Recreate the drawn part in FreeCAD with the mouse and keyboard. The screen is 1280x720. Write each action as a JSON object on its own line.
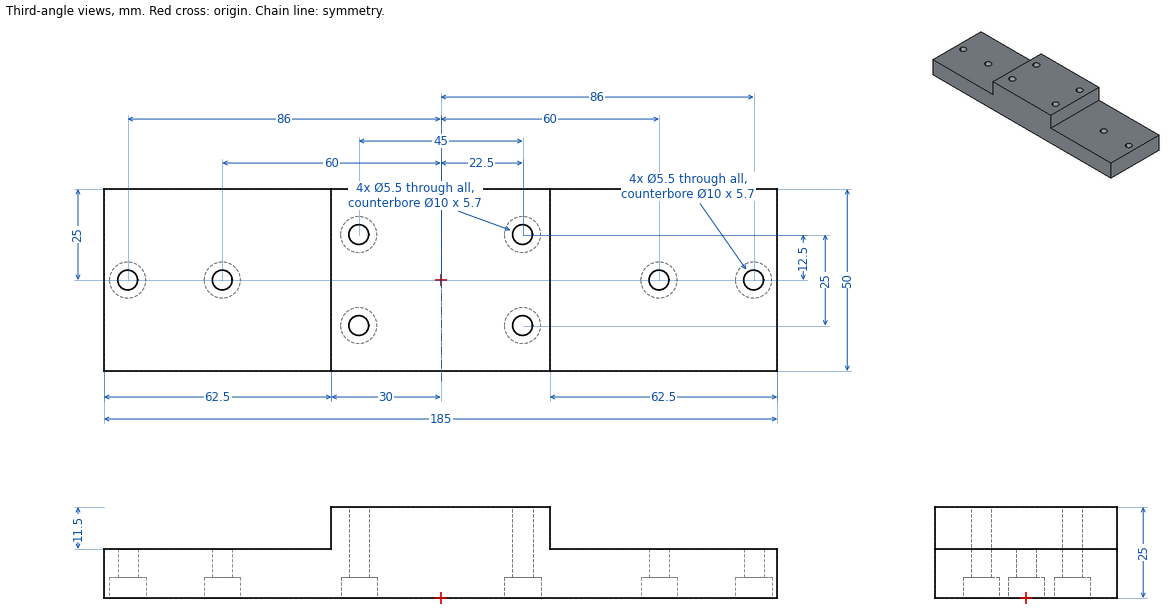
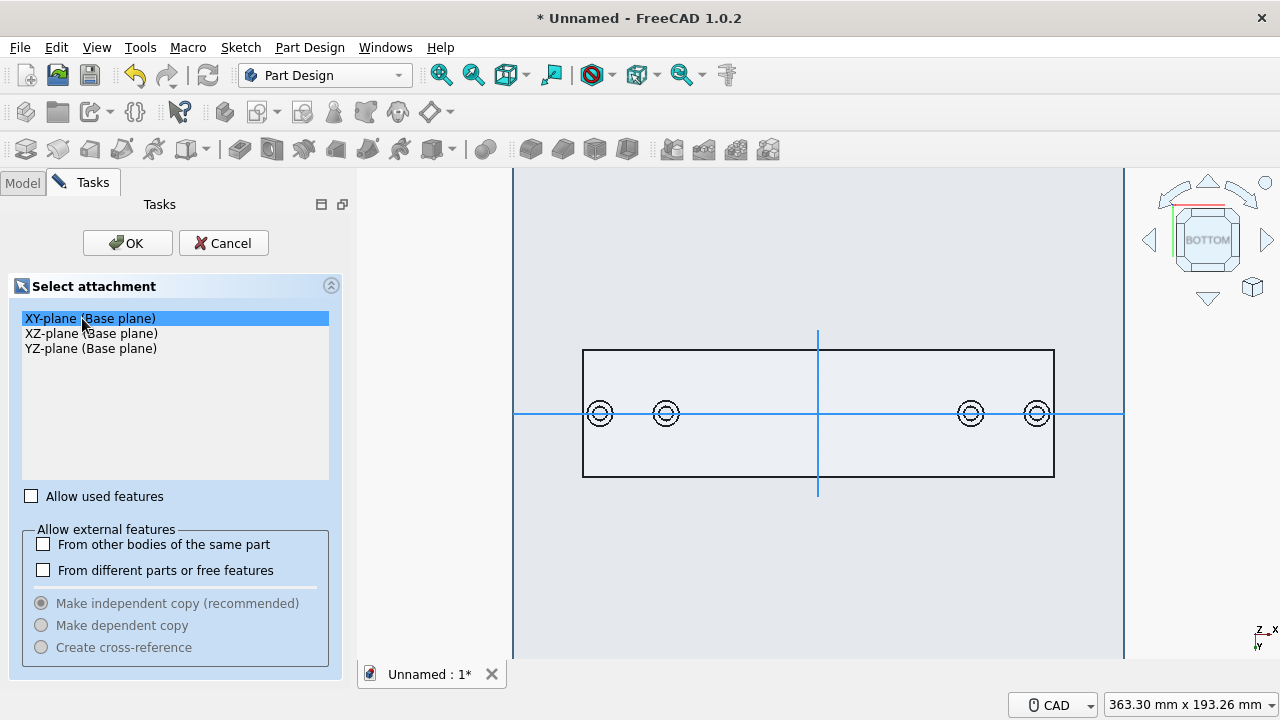
{"action": "left_click", "coordinate": [128, 243]}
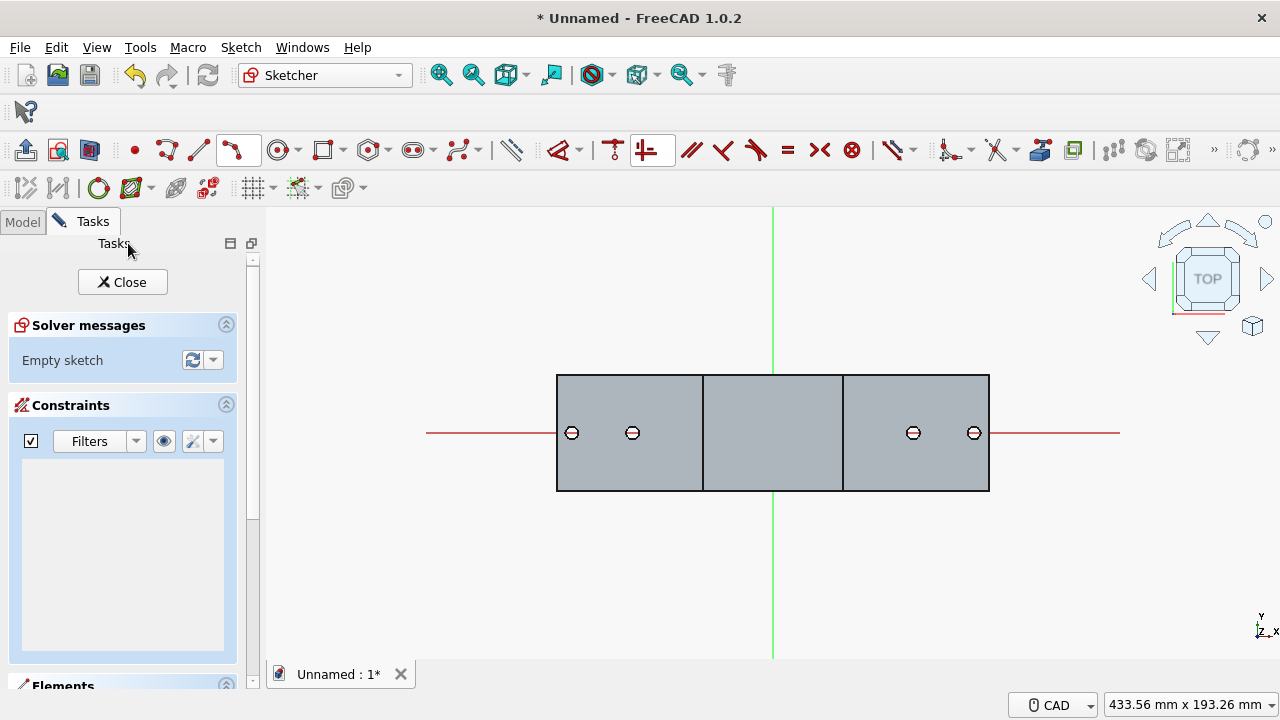
{"action": "left_click", "coordinate": [90, 150]}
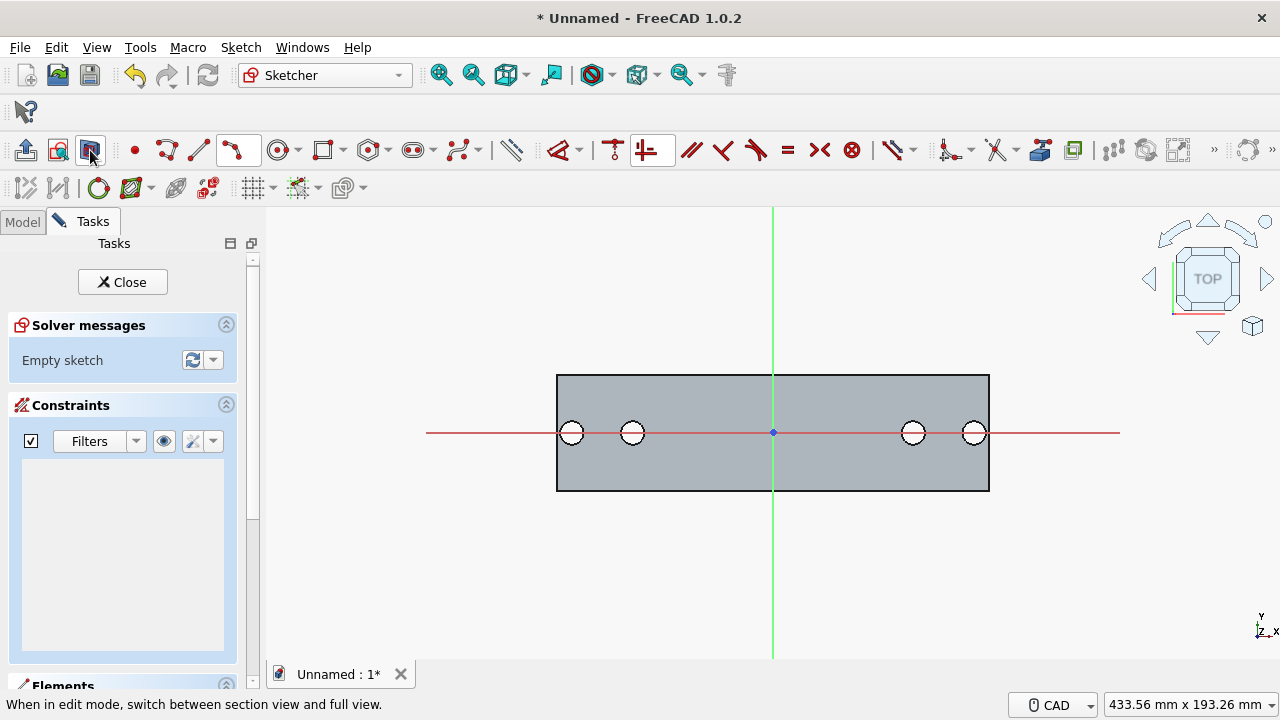
{"action": "scroll", "coordinate": [795, 433], "scroll_direction": "up", "scroll_amount": 7}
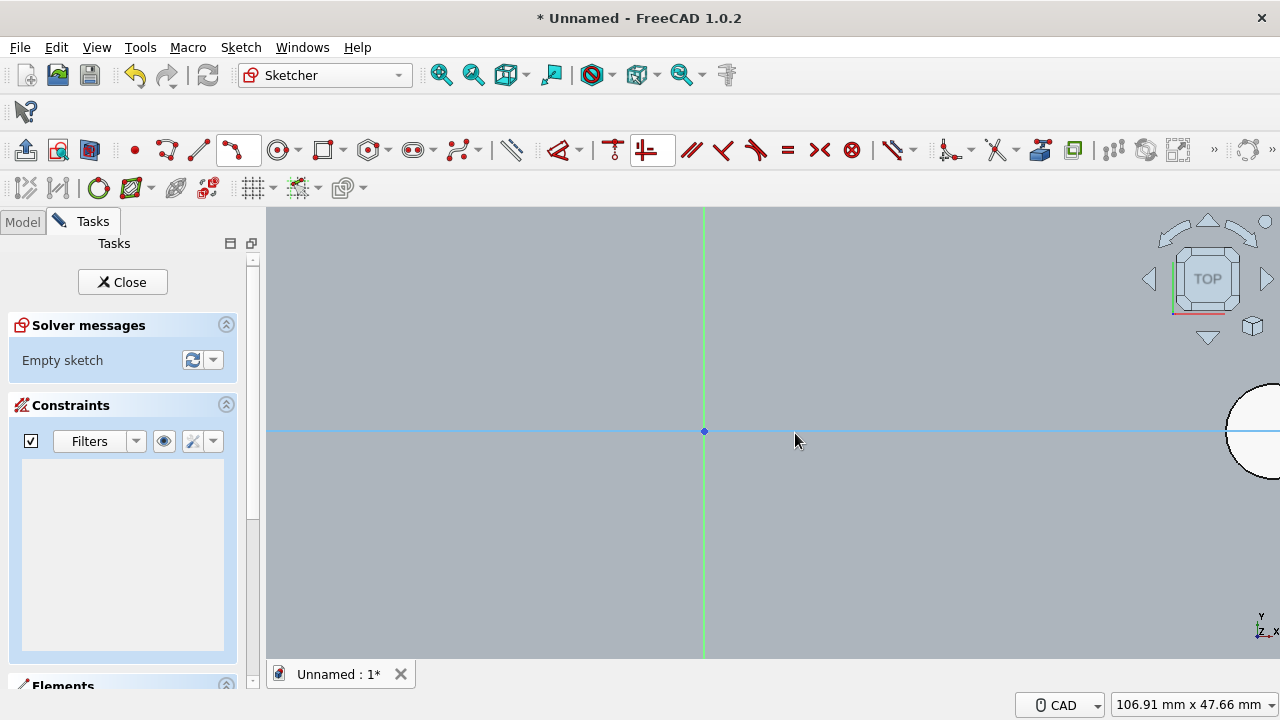
{"action": "left_click", "coordinate": [278, 150]}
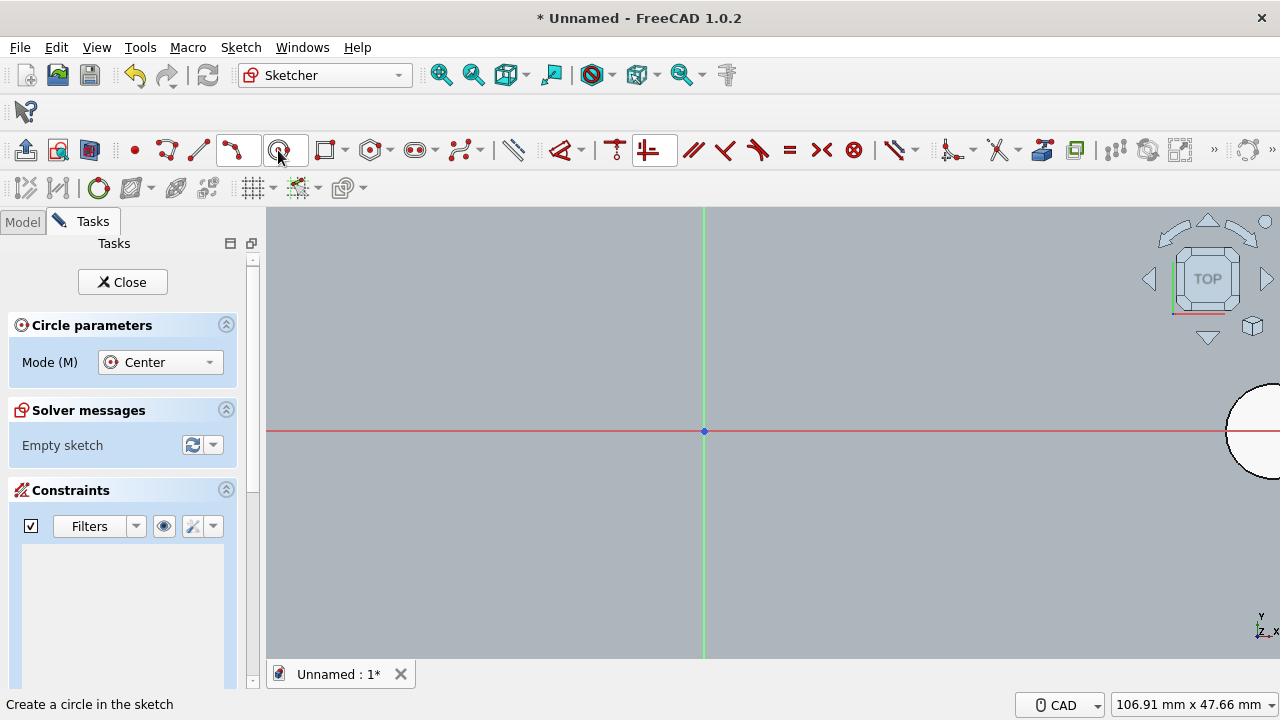
{"action": "left_click", "coordinate": [918, 313]}
{"action": "mouse_move", "coordinate": [936, 294]}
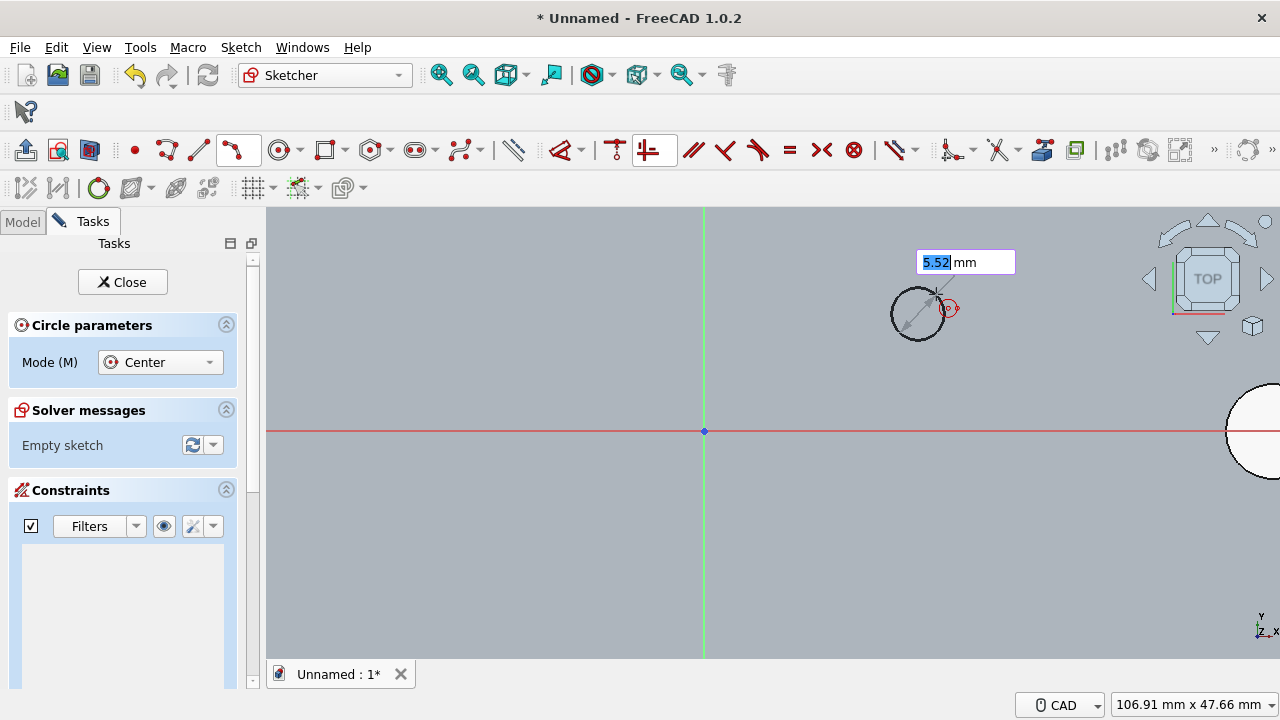
{"action": "type", "text": "5.5"}
{"action": "key", "text": "Return"}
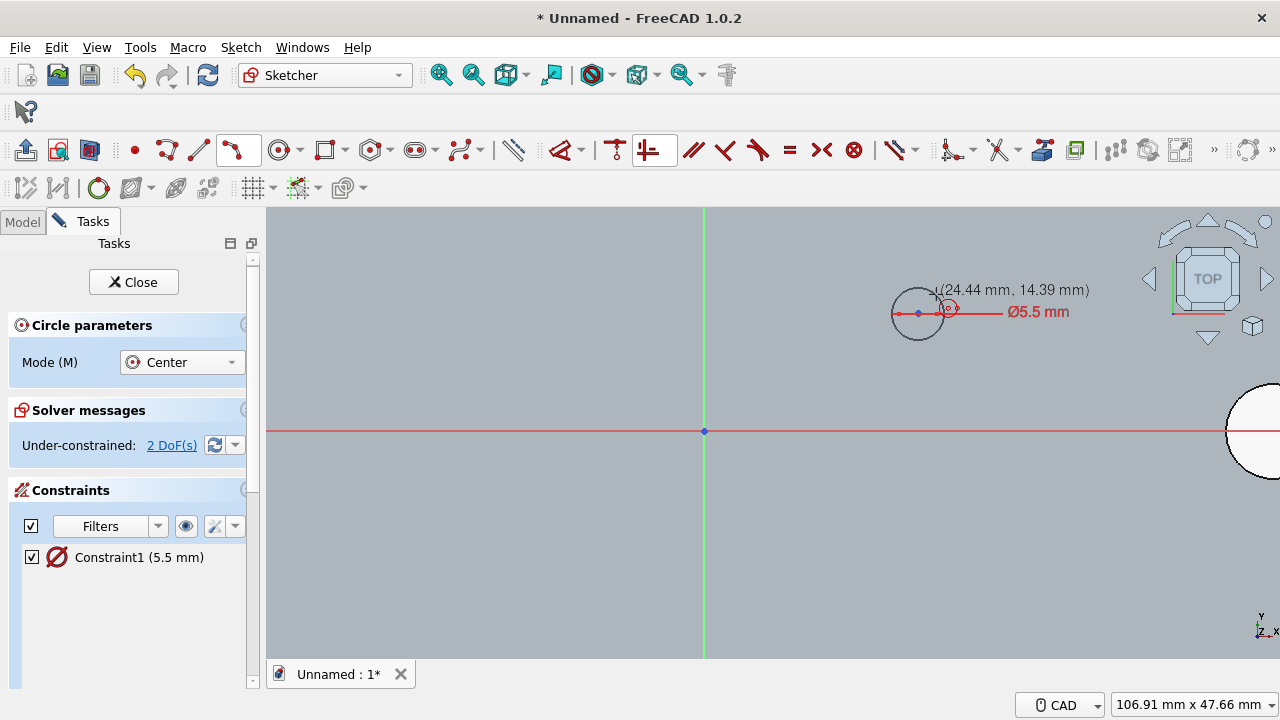
{"action": "left_click", "coordinate": [918, 550]}
{"action": "mouse_move", "coordinate": [936, 532]}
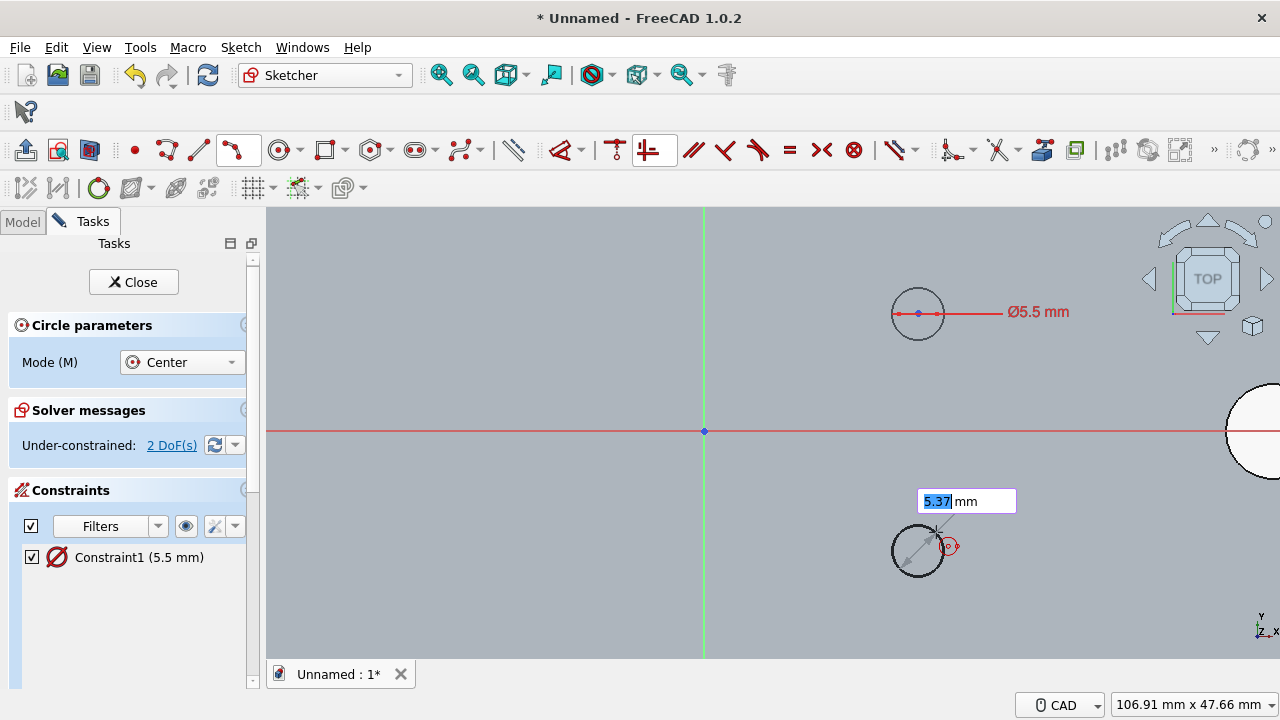
{"action": "type", "text": "5.5"}
{"action": "key", "text": "Return"}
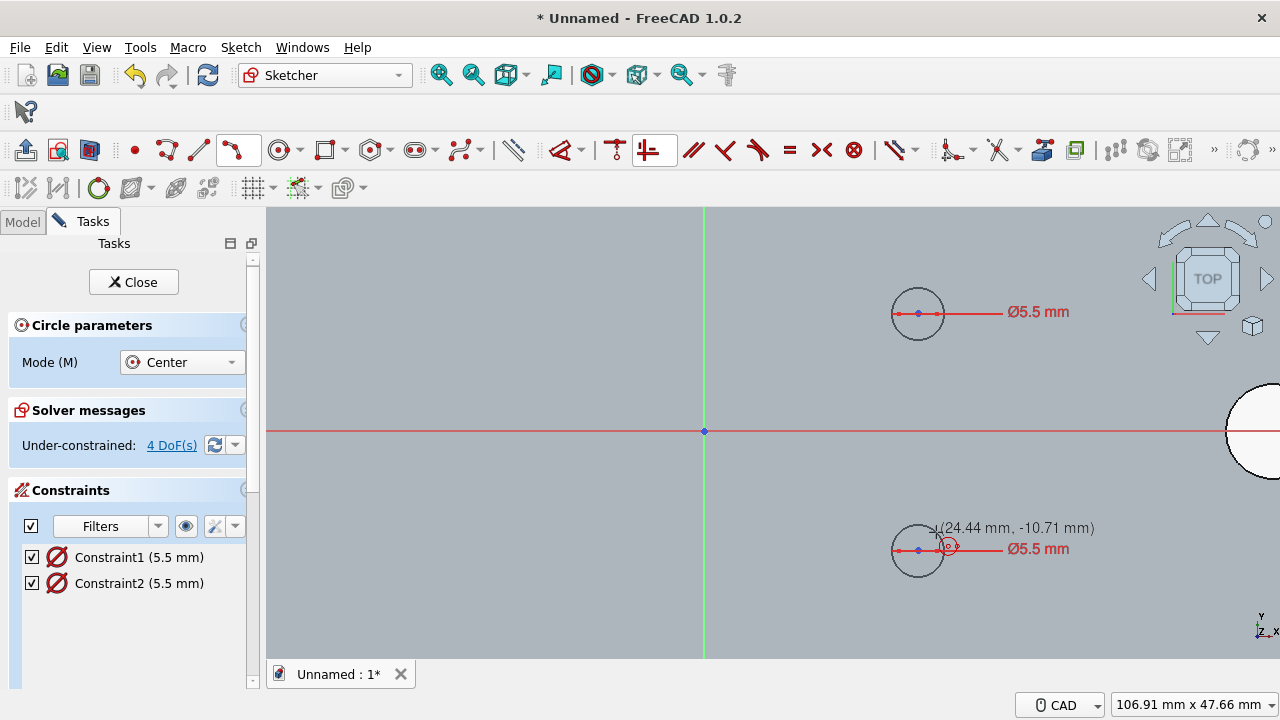
{"action": "left_click", "coordinate": [491, 313]}
{"action": "mouse_move", "coordinate": [509, 294]}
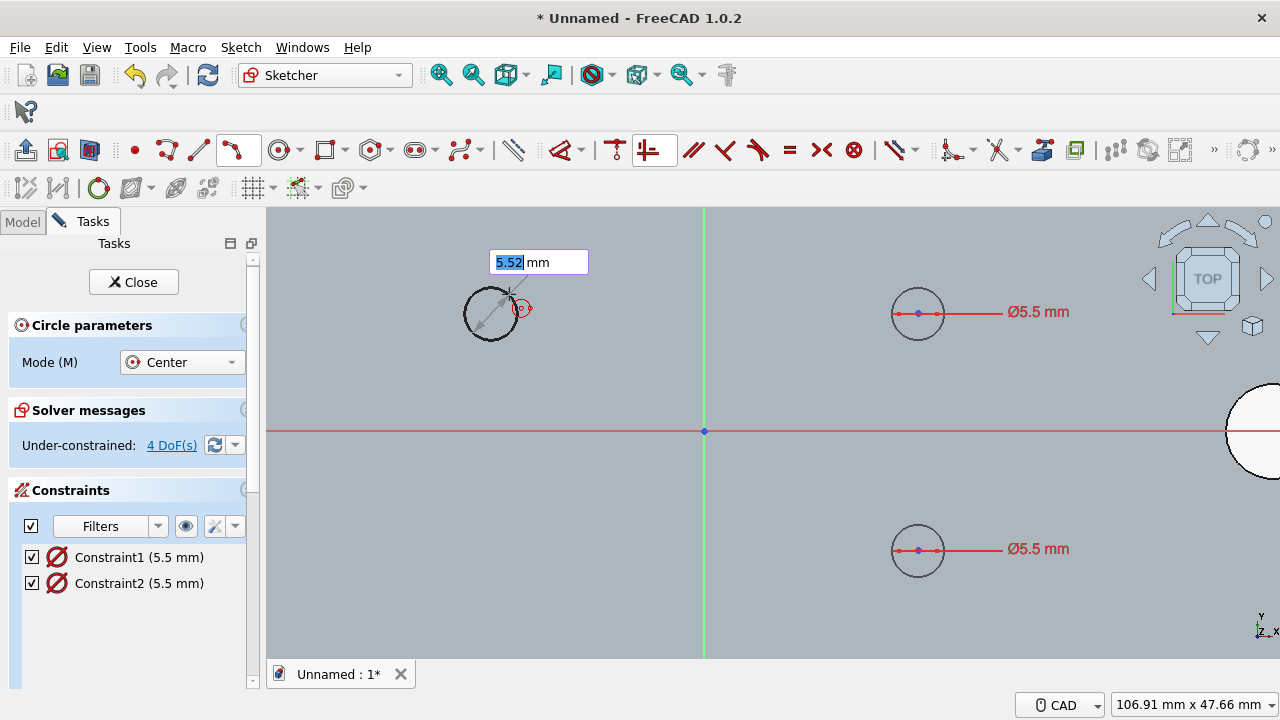
{"action": "type", "text": "5.5"}
{"action": "key", "text": "Return"}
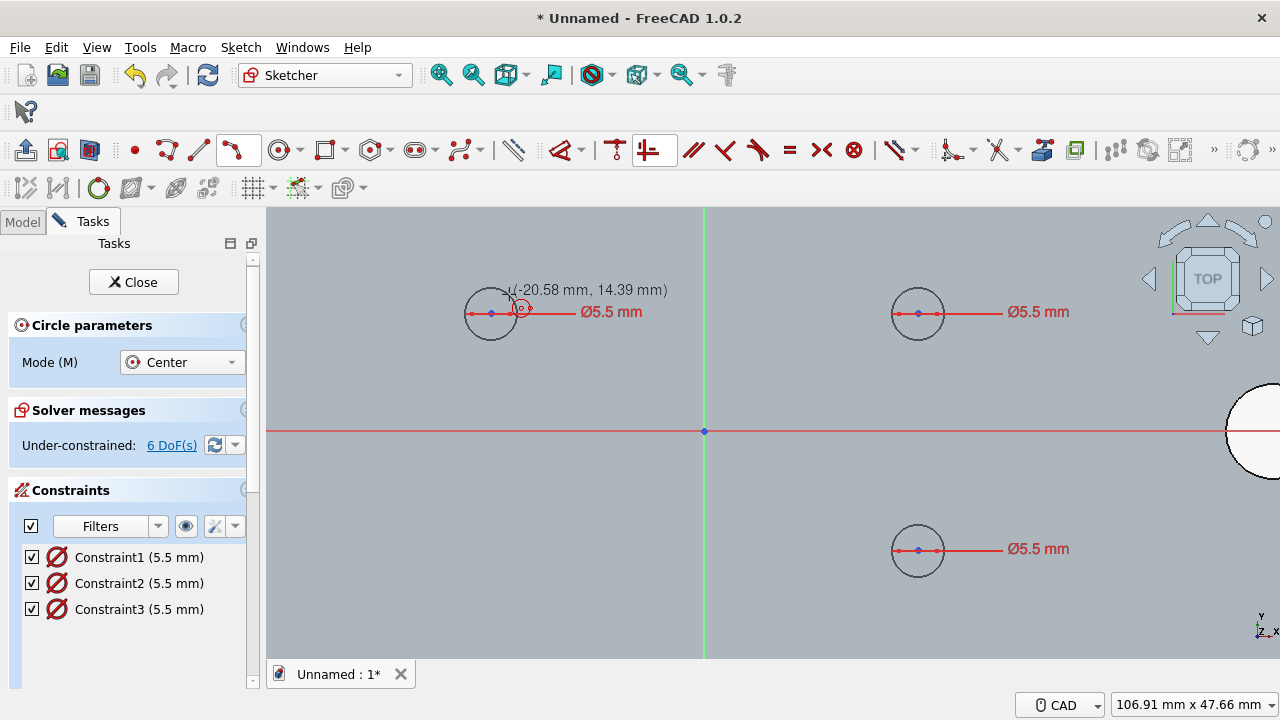
{"action": "left_click", "coordinate": [491, 550]}
{"action": "mouse_move", "coordinate": [509, 532]}